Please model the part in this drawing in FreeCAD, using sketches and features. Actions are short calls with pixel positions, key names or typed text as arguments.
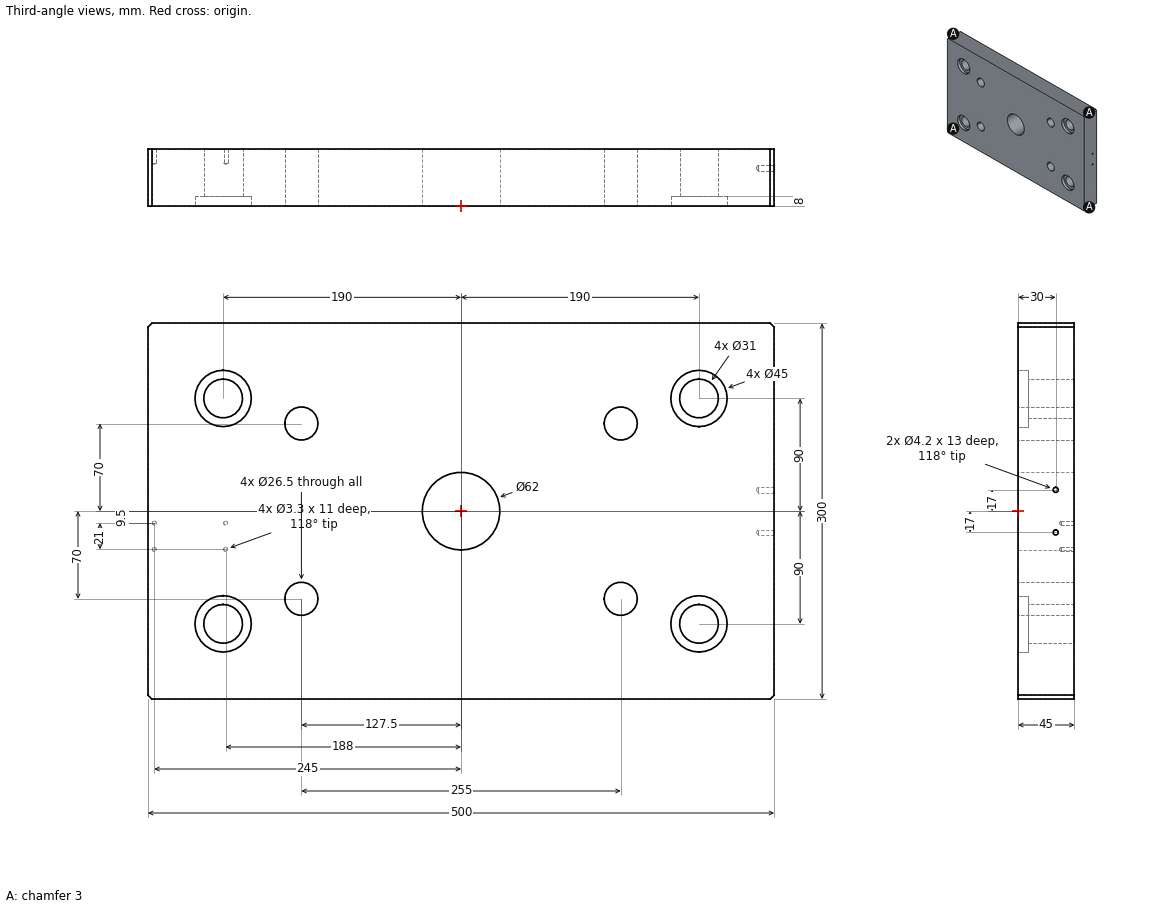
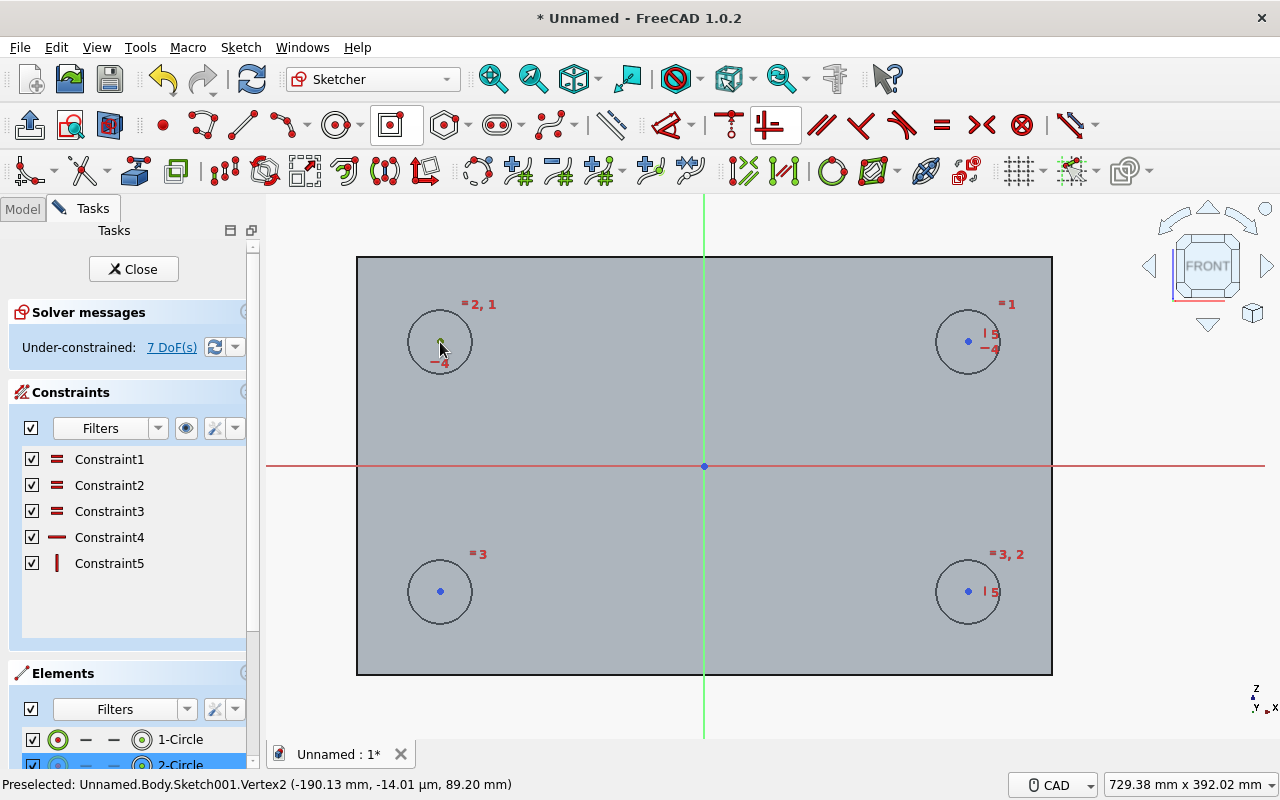
click(440, 592)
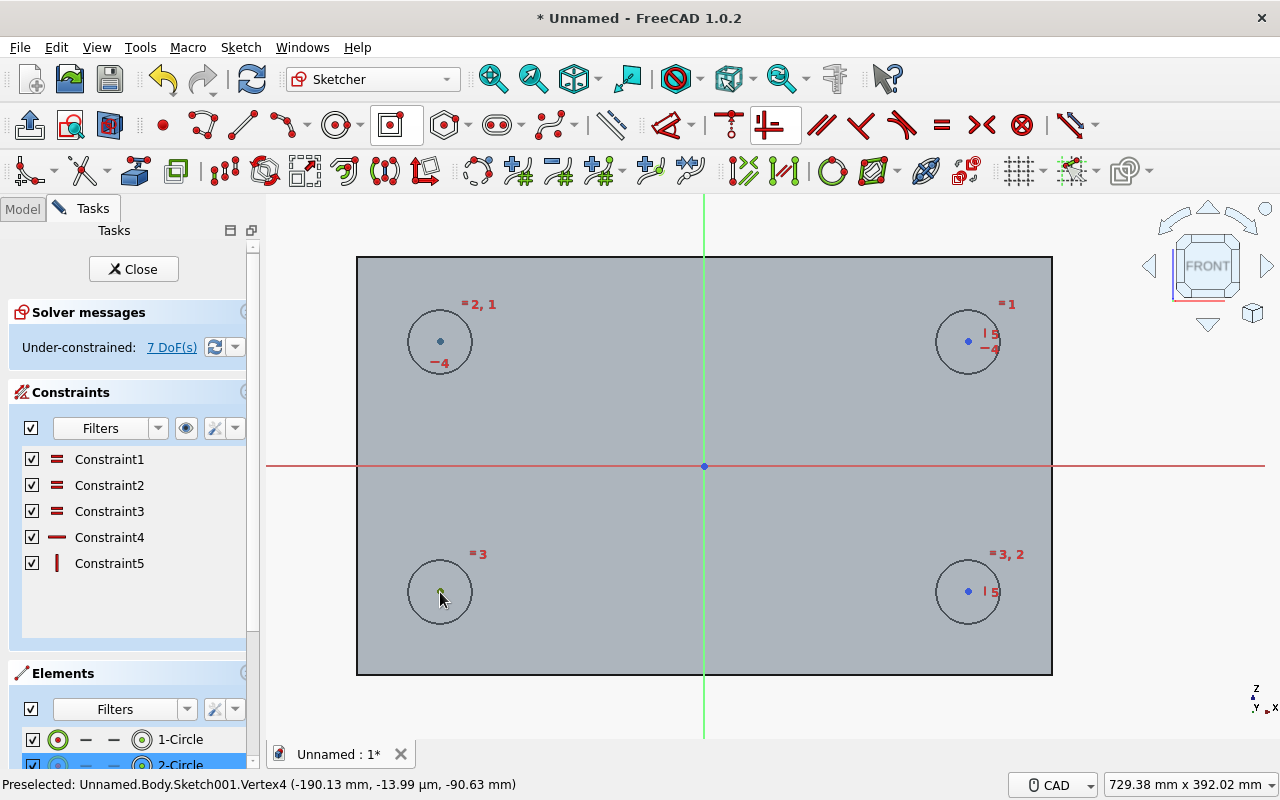
click(796, 126)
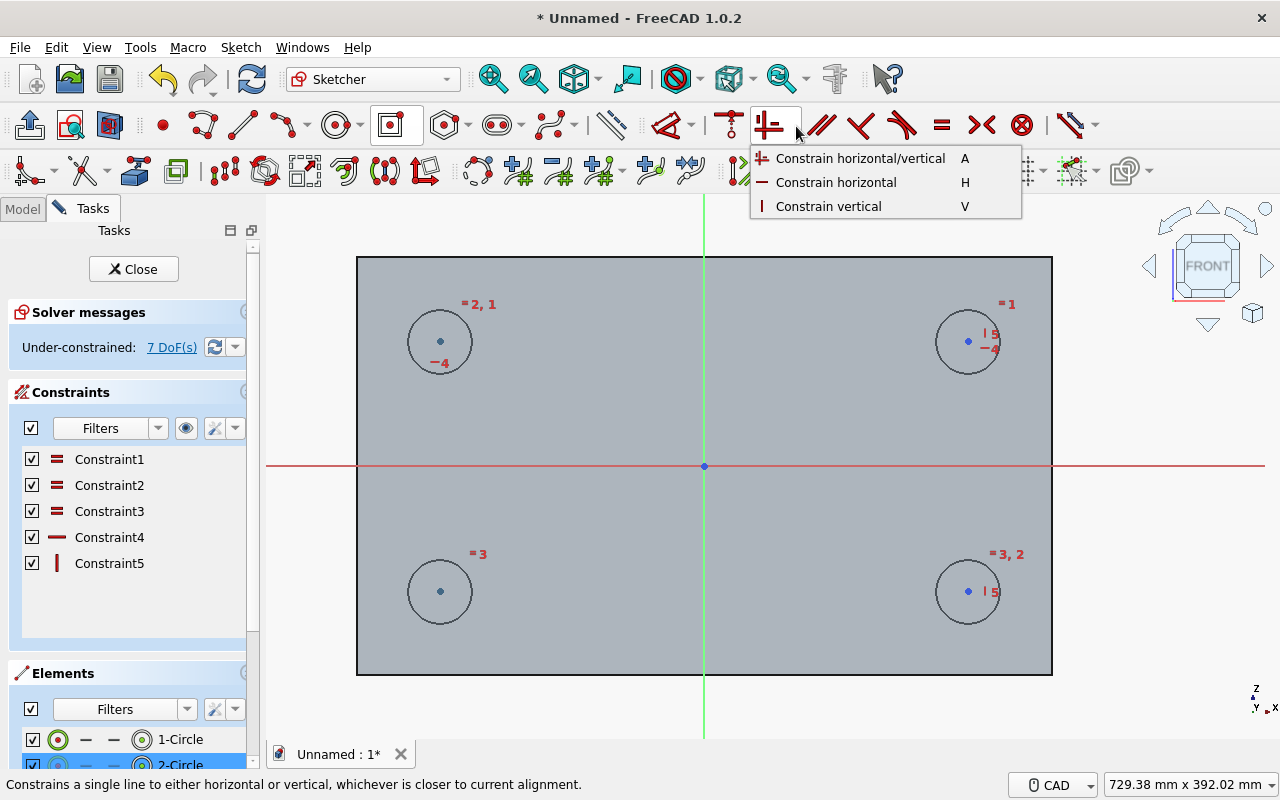
click(886, 206)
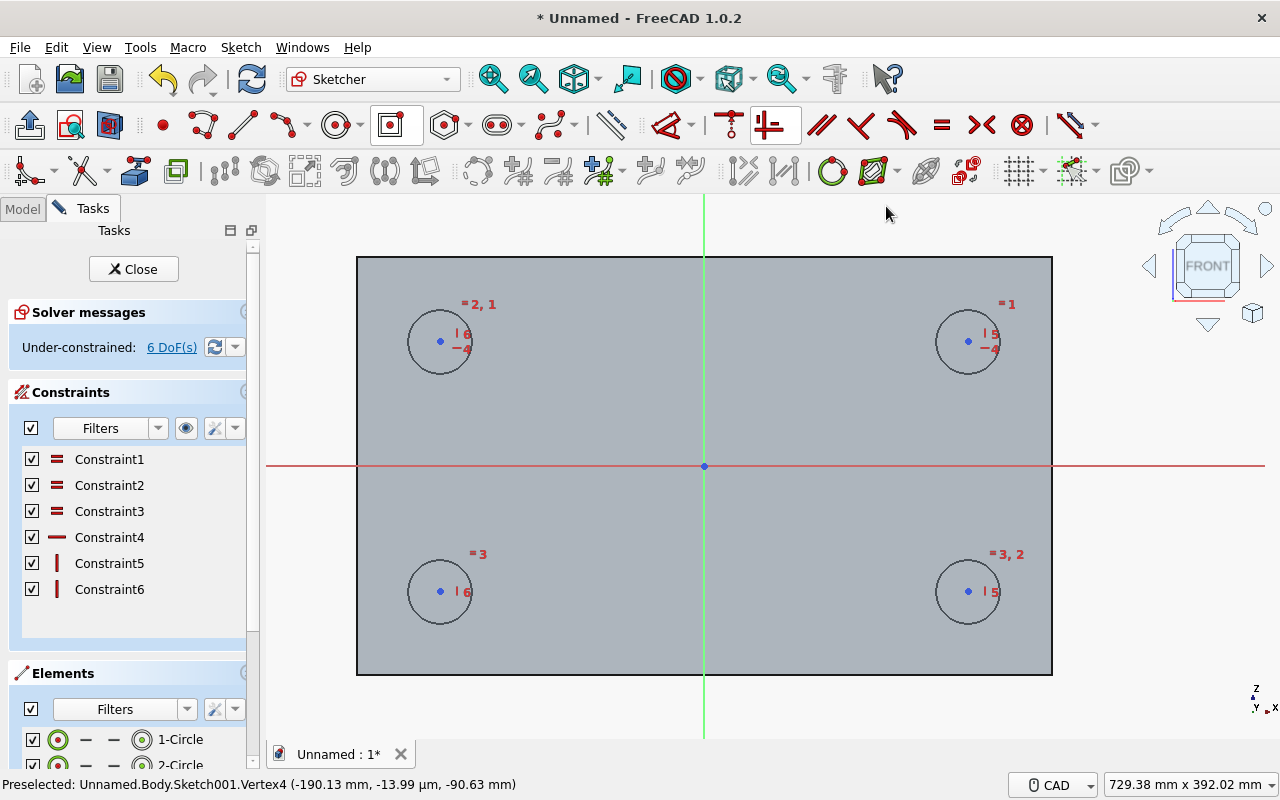
click(968, 592)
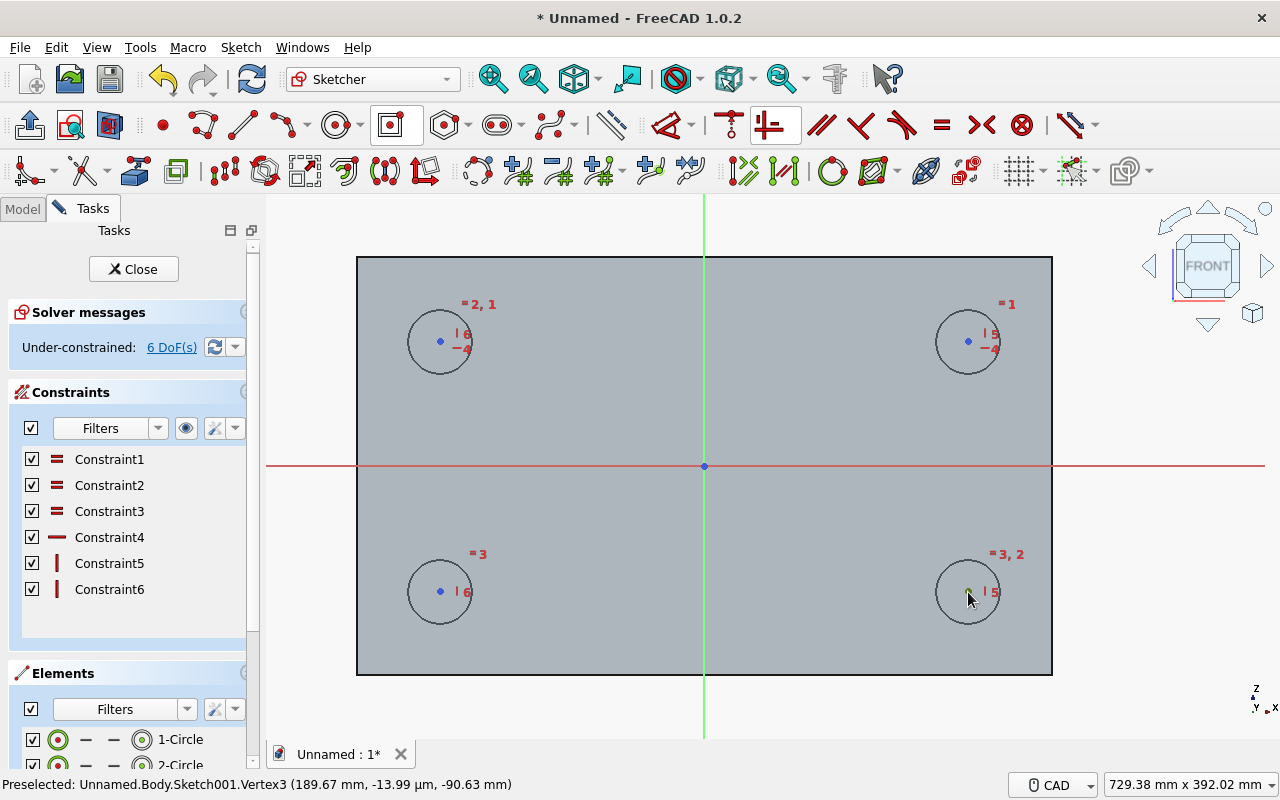
click(440, 592)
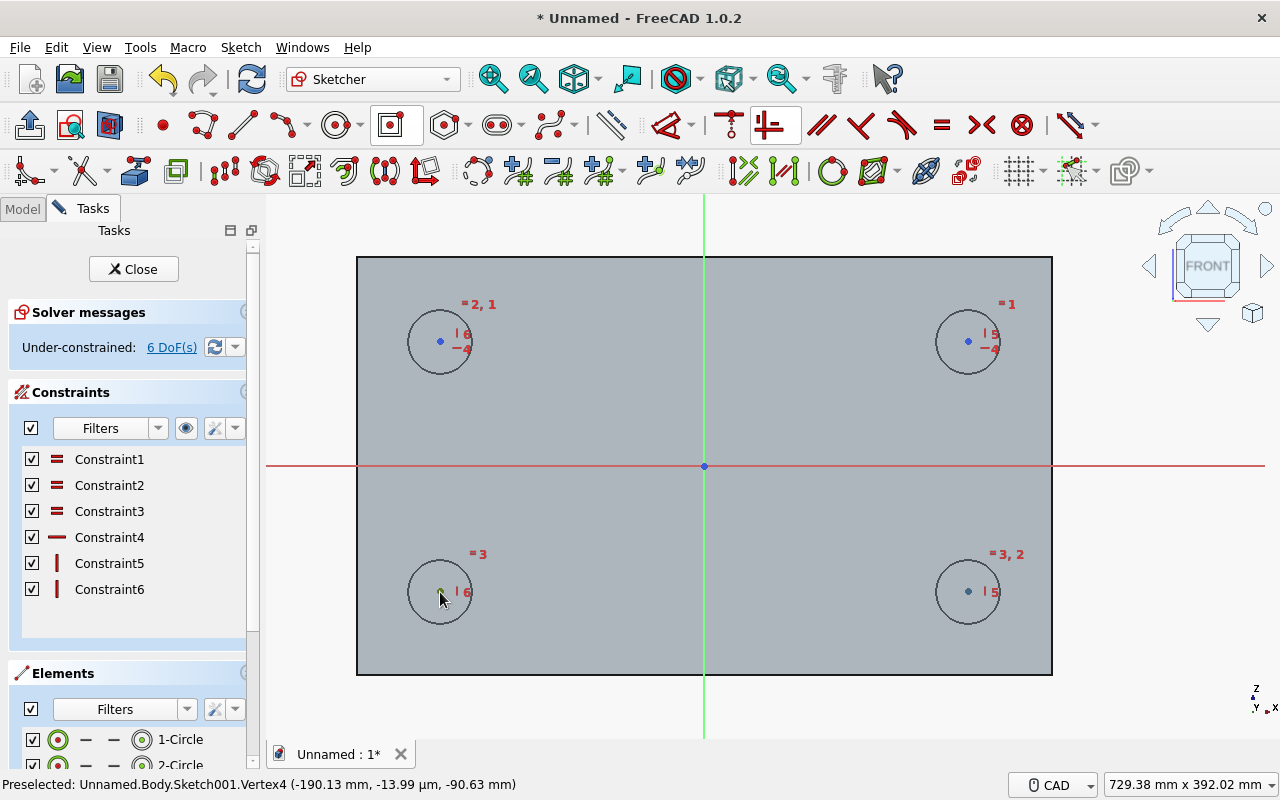
key(h)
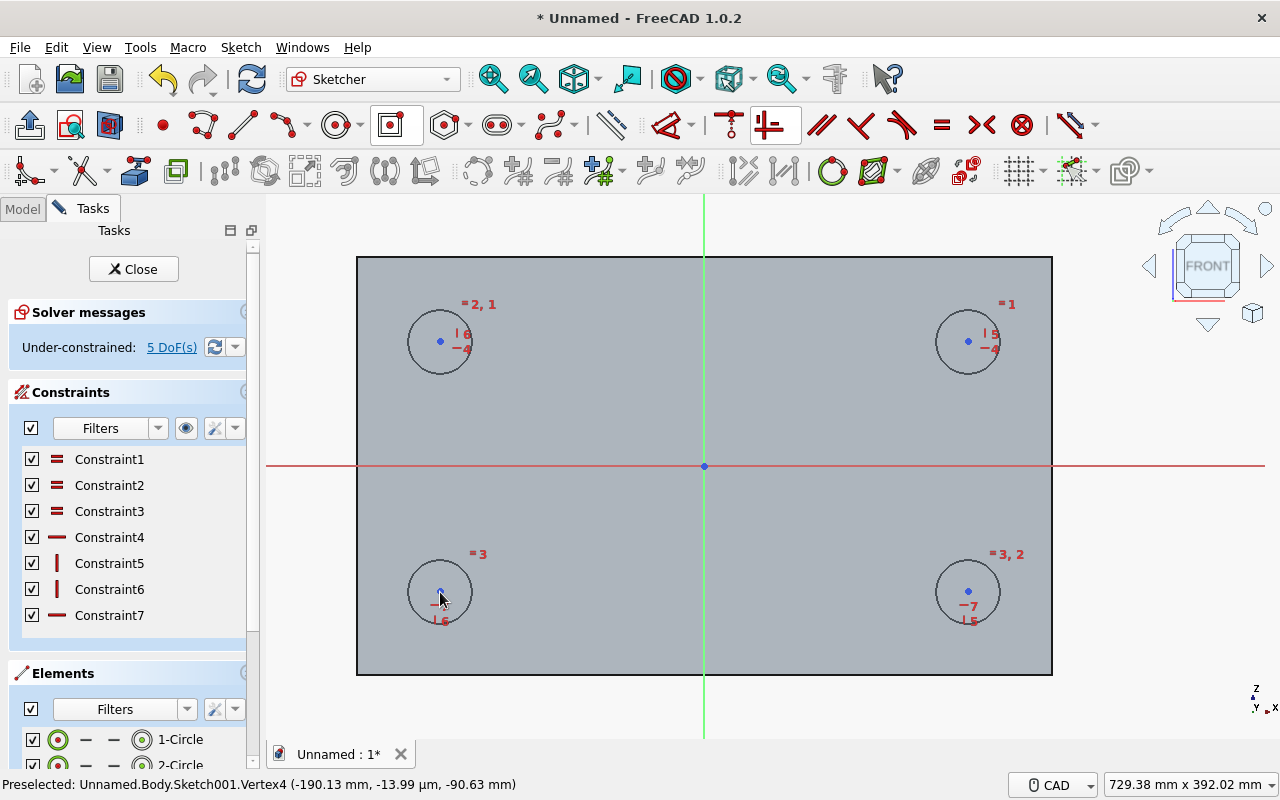
click(666, 126)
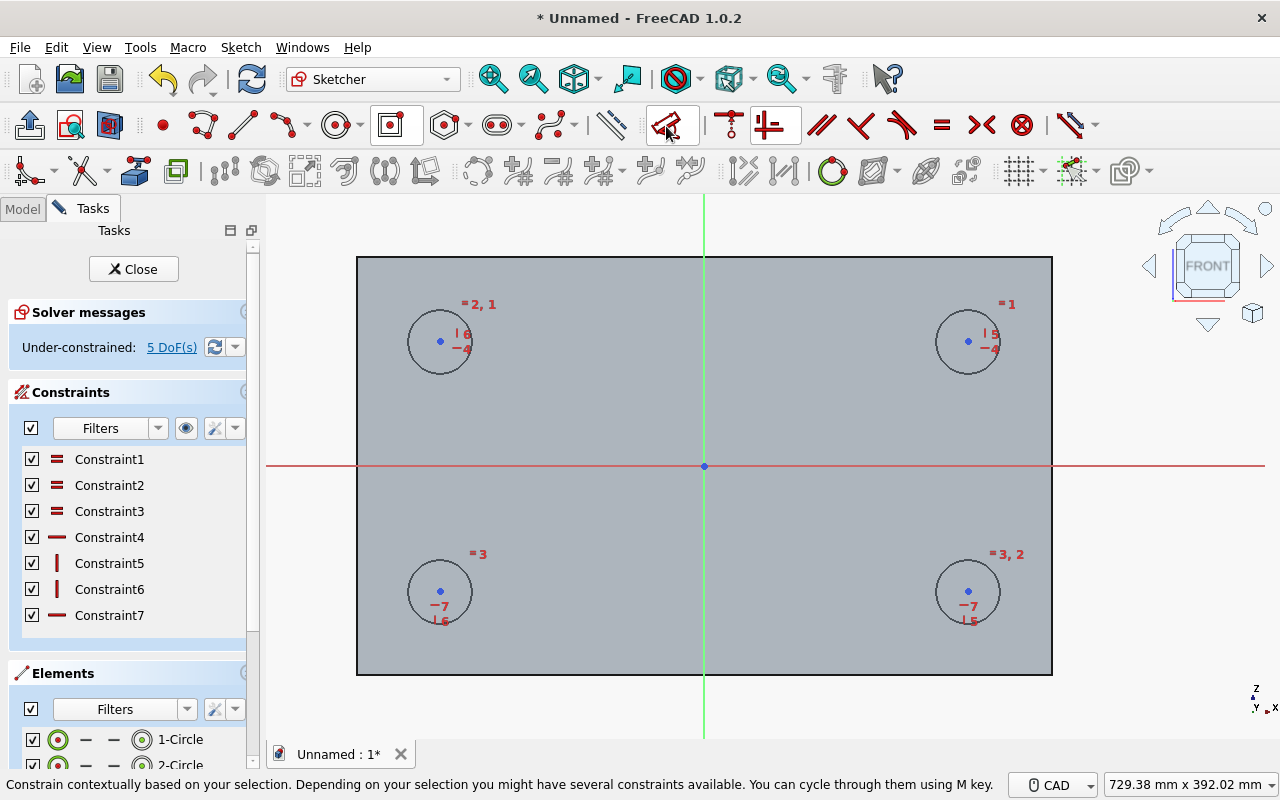
click(990, 319)
click(1012, 296)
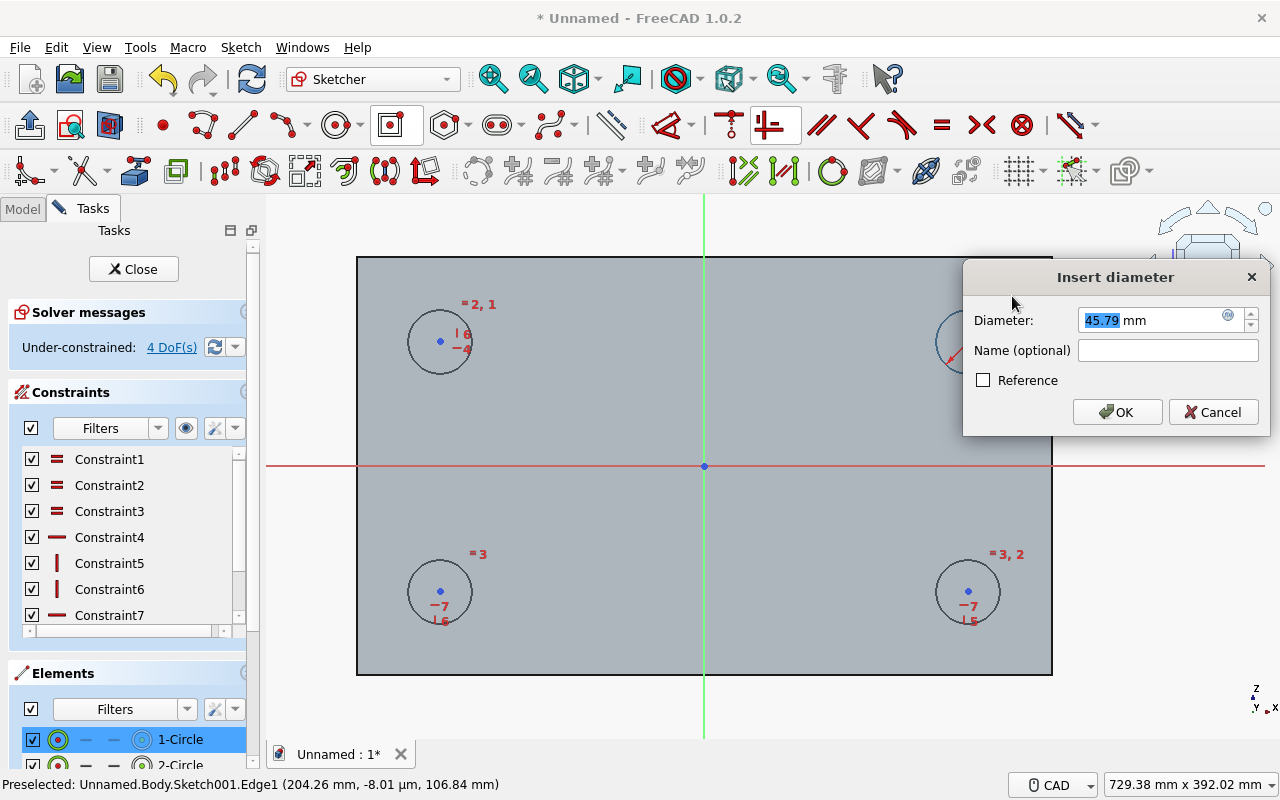
text(45)
key(Return)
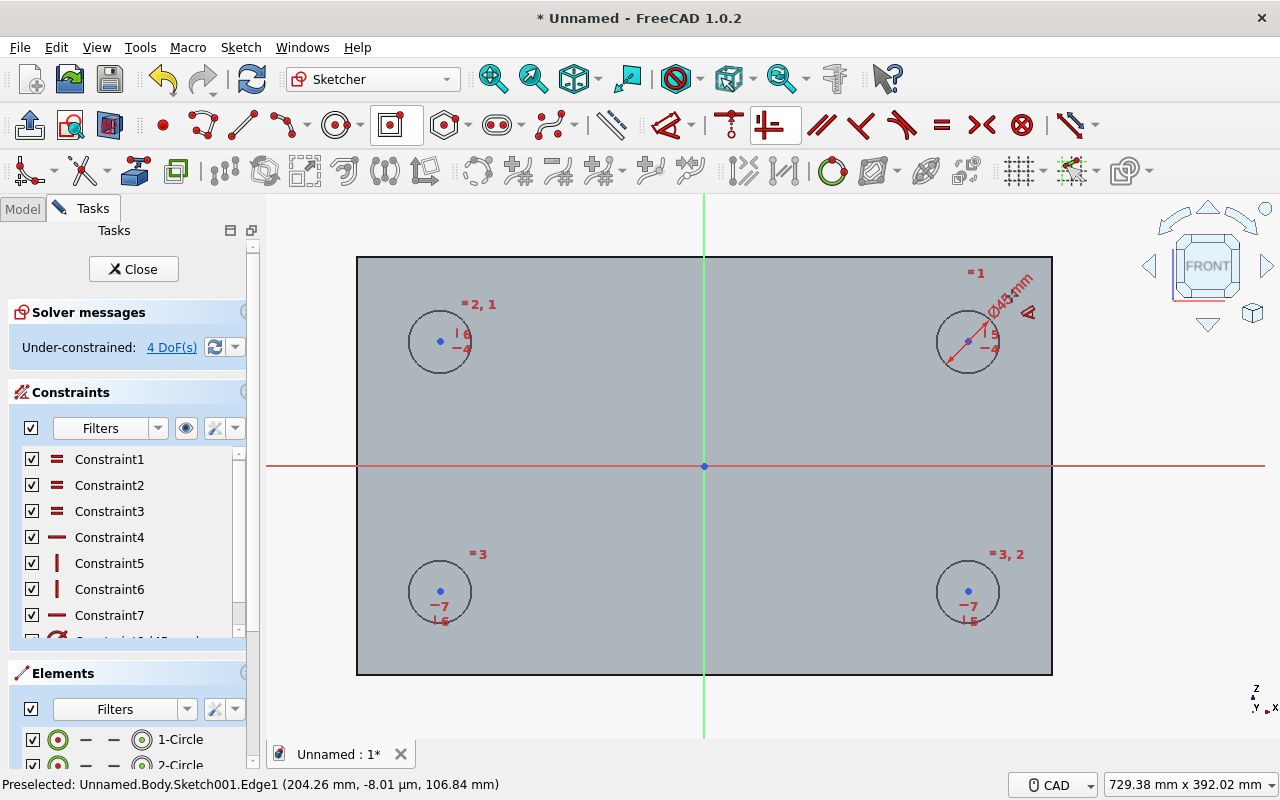
click(968, 342)
click(1002, 404)